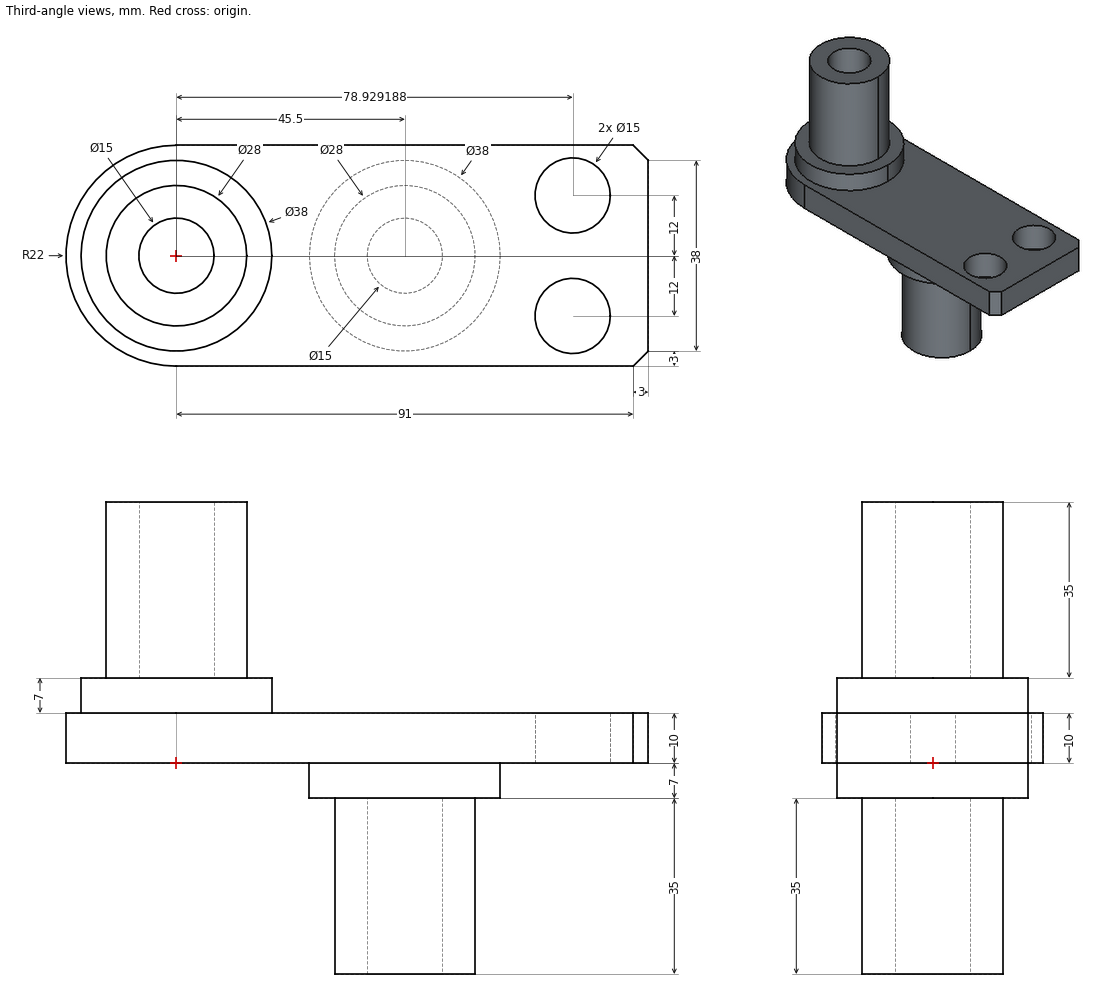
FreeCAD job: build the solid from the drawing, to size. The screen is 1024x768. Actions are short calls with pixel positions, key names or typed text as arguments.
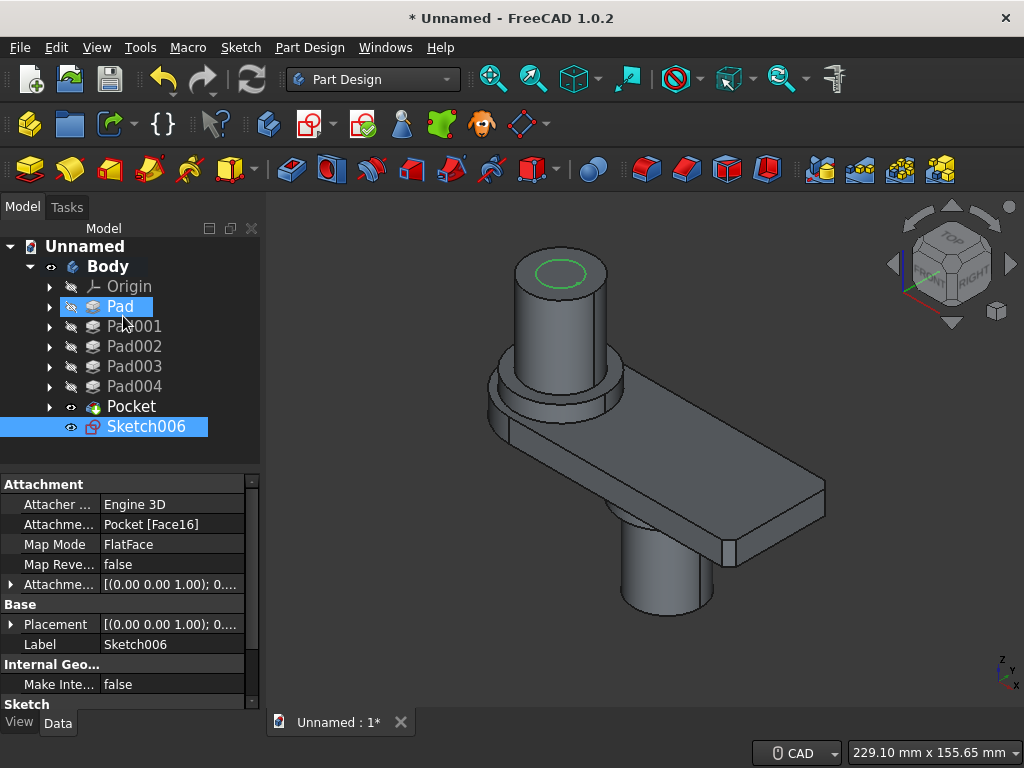
click(292, 170)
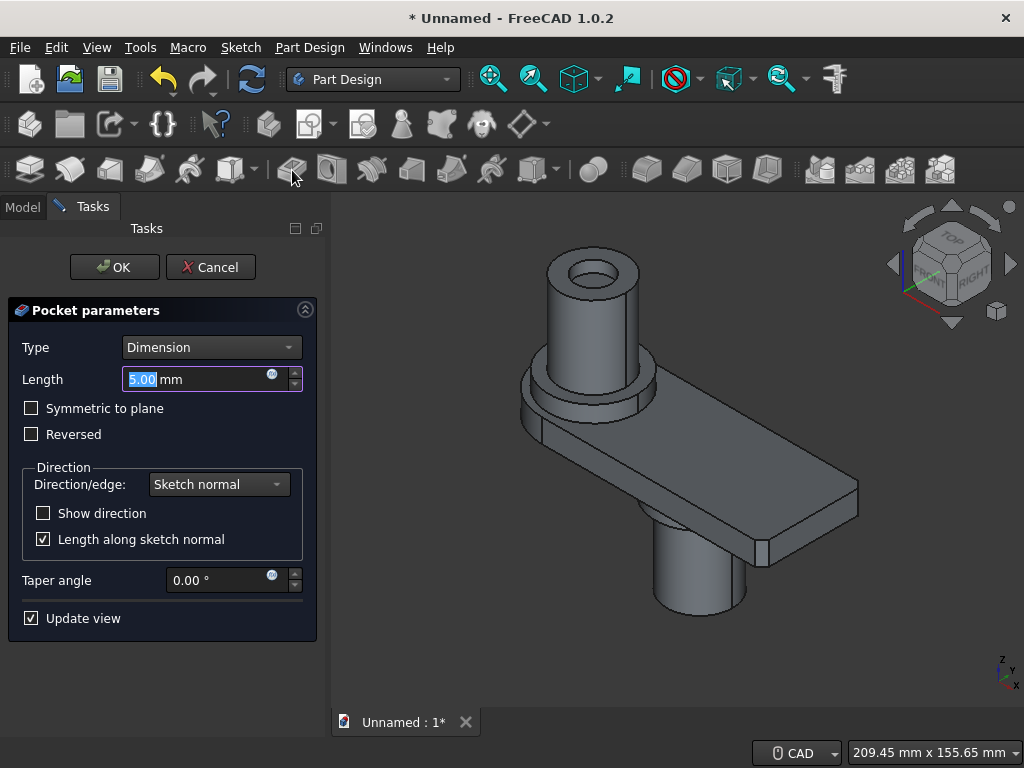
text(35)
key(Tab)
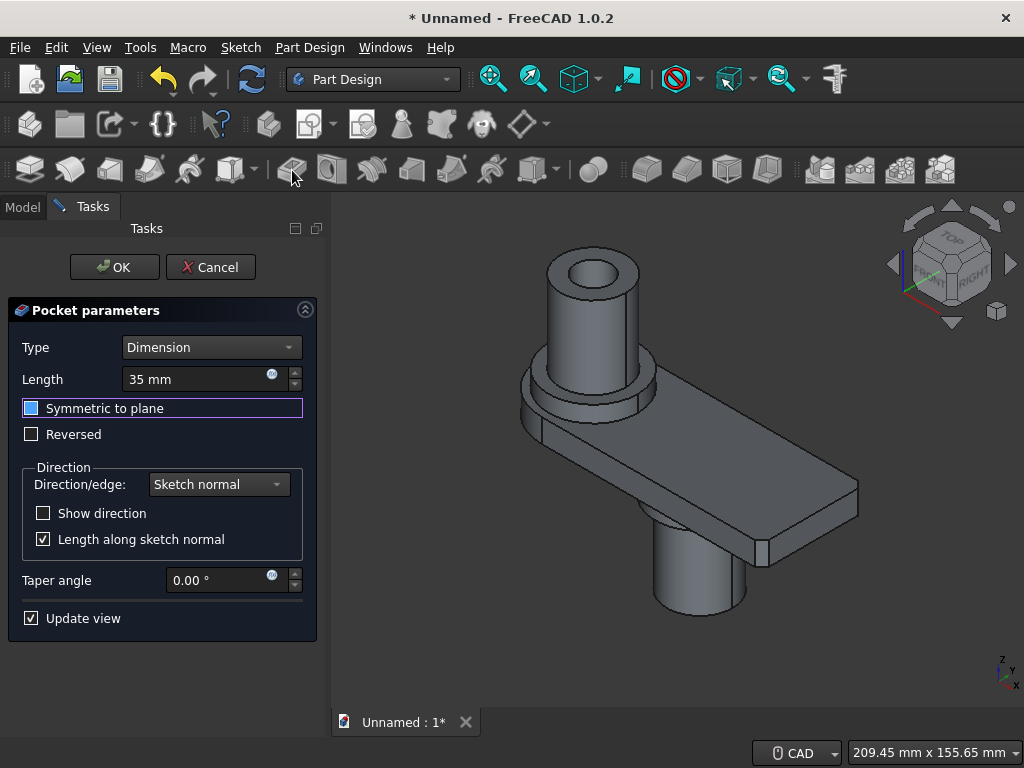
click(115, 267)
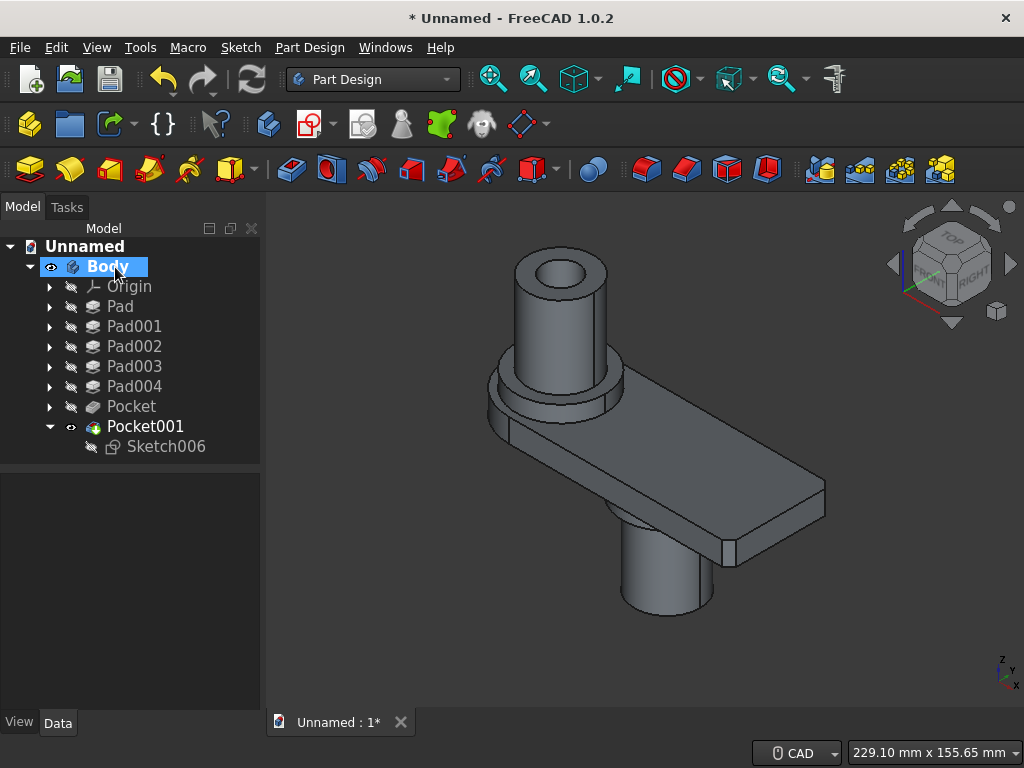
click(723, 480)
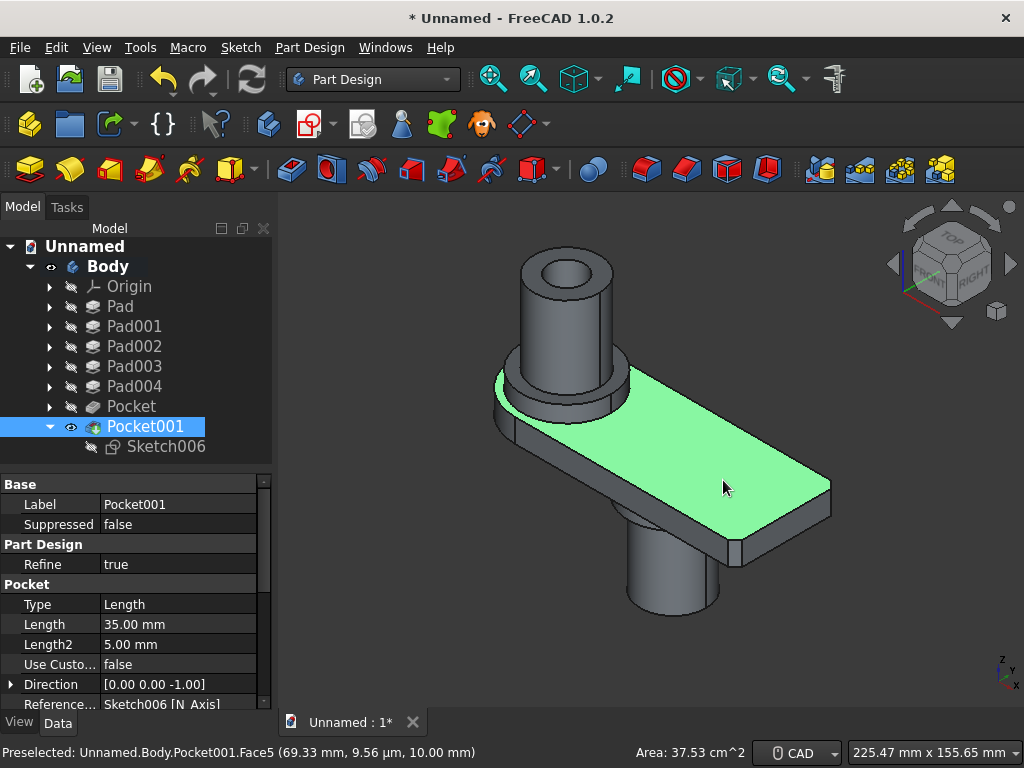
click(310, 124)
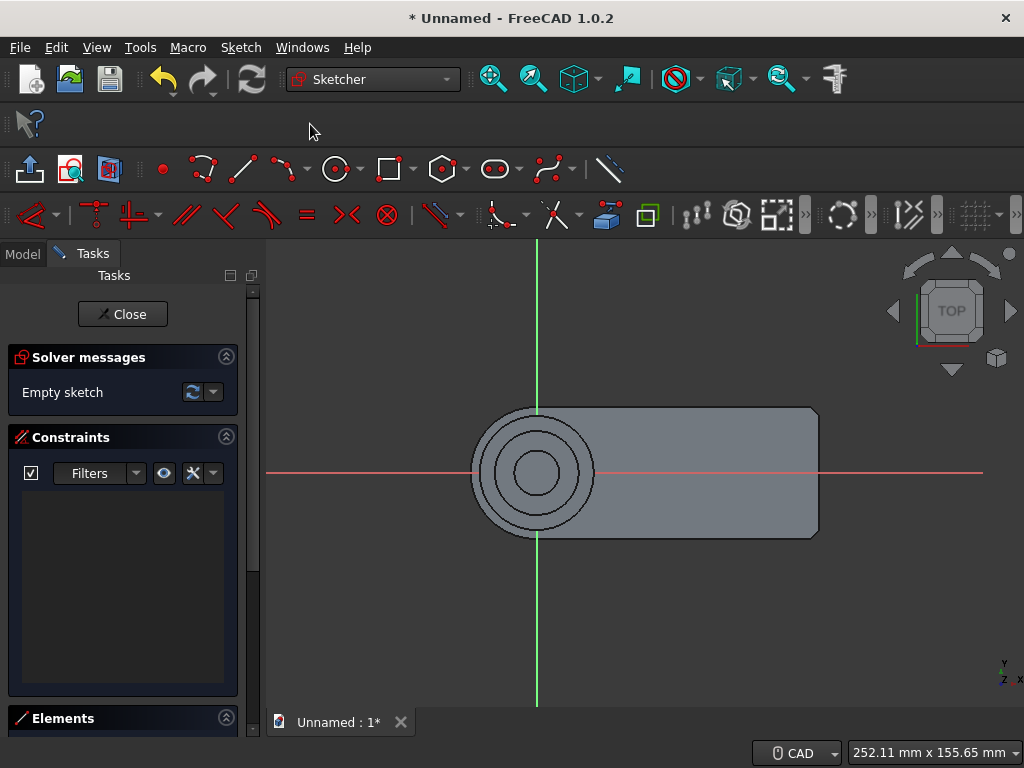
scroll(850, 473, up, 2)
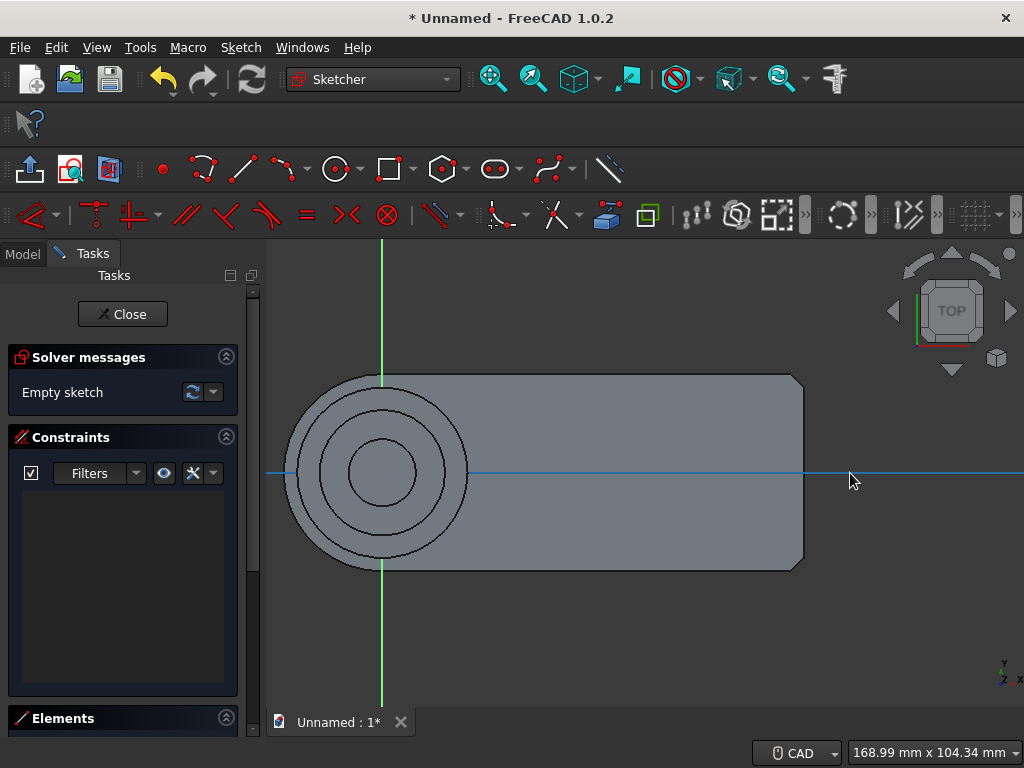
click(336, 170)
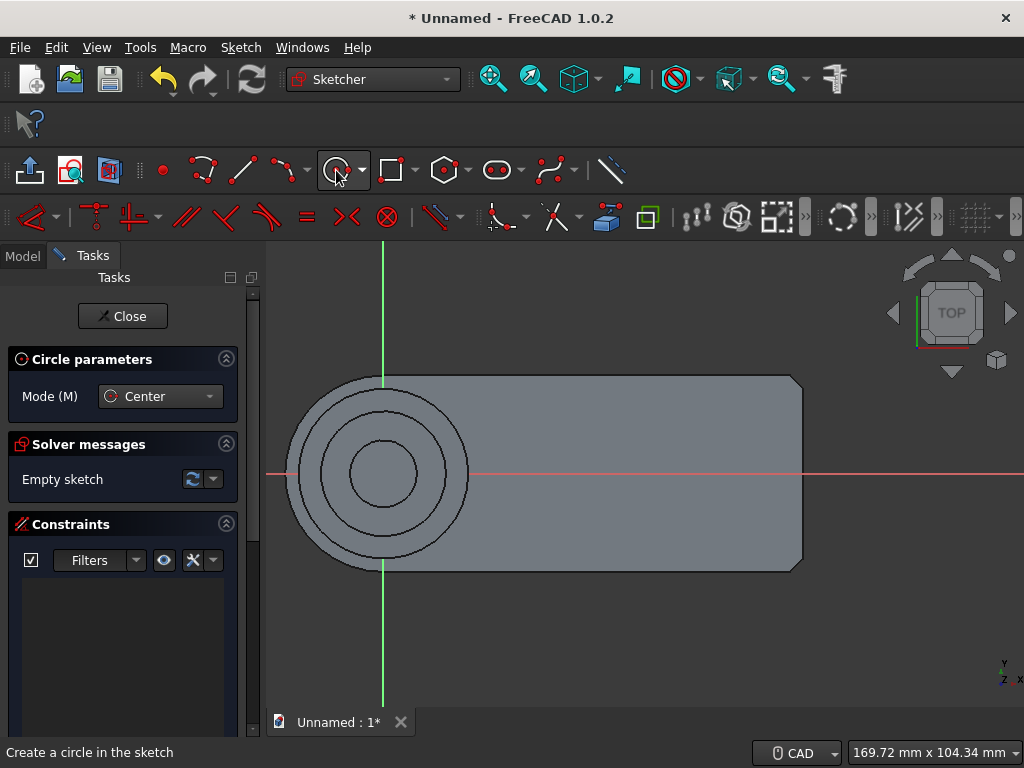
click(736, 420)
move(760, 396)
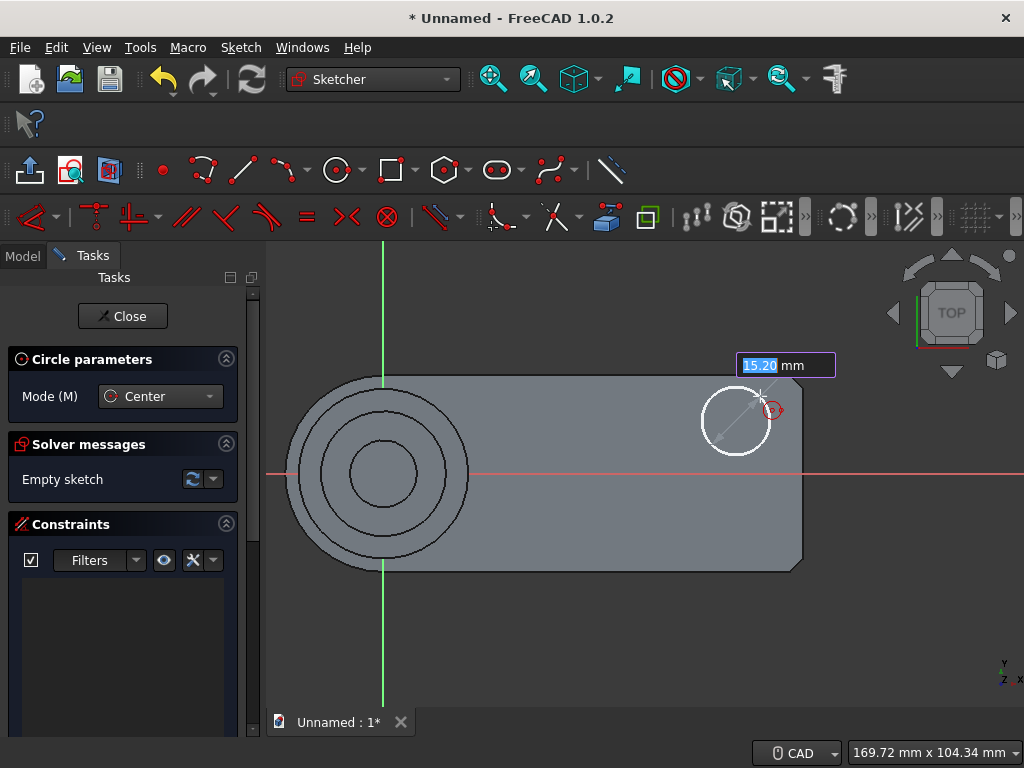
text(15)
key(Return)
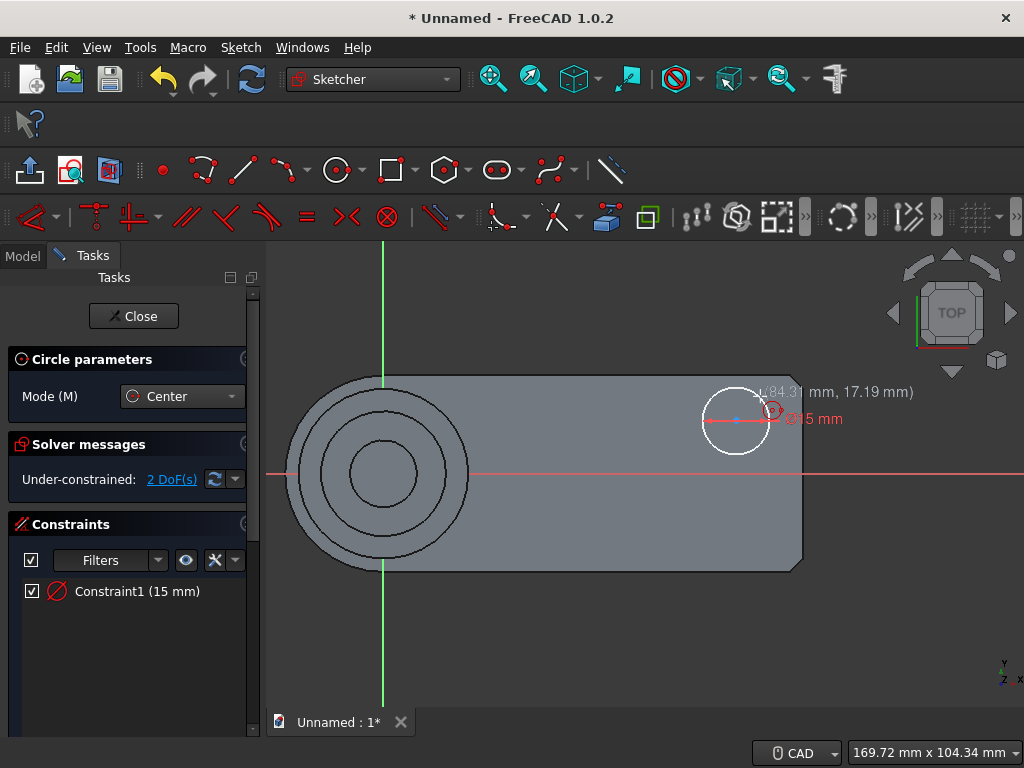
click(736, 527)
move(760, 504)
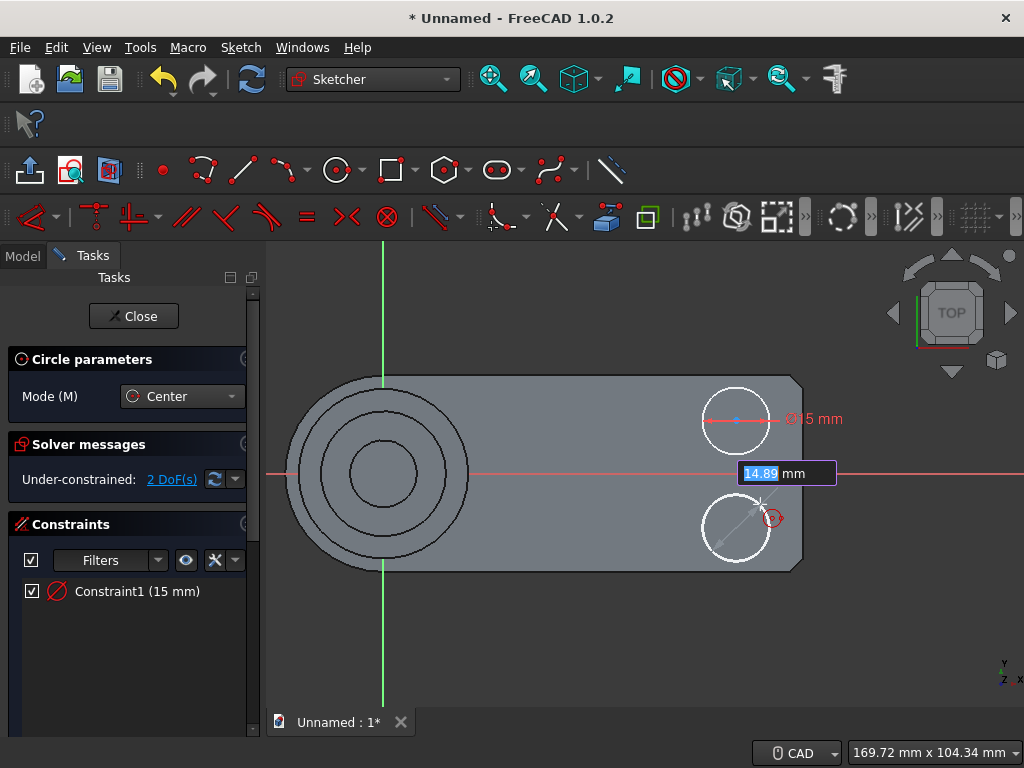
text(15)
key(Return)
key(Escape)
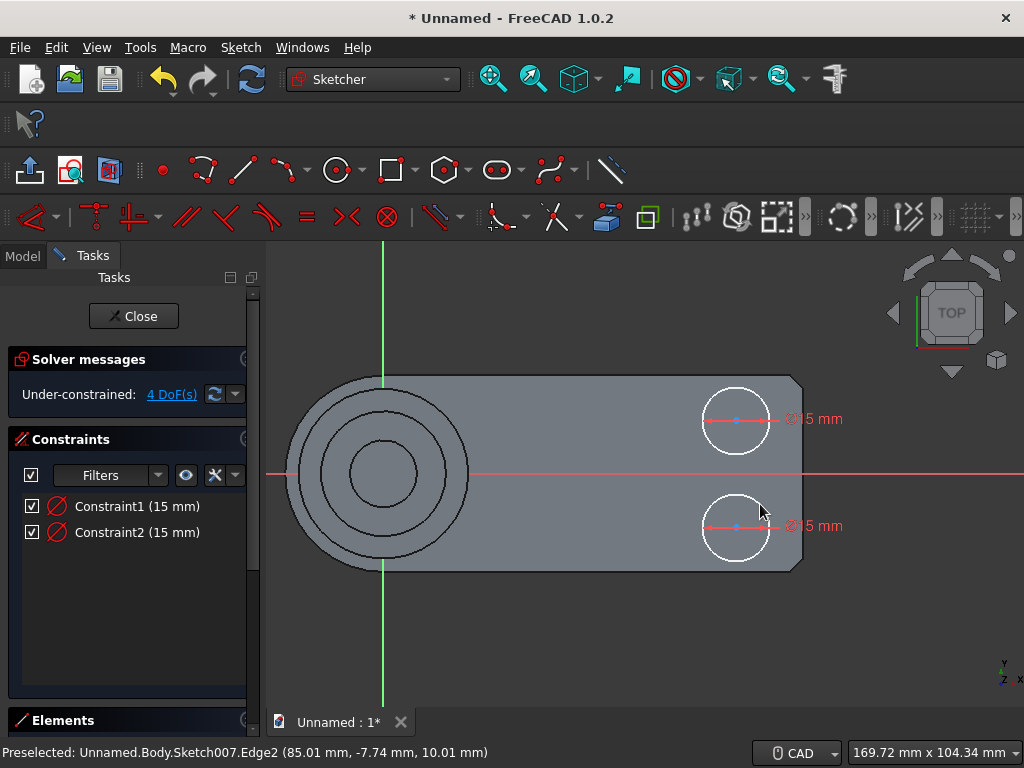
click(736, 421)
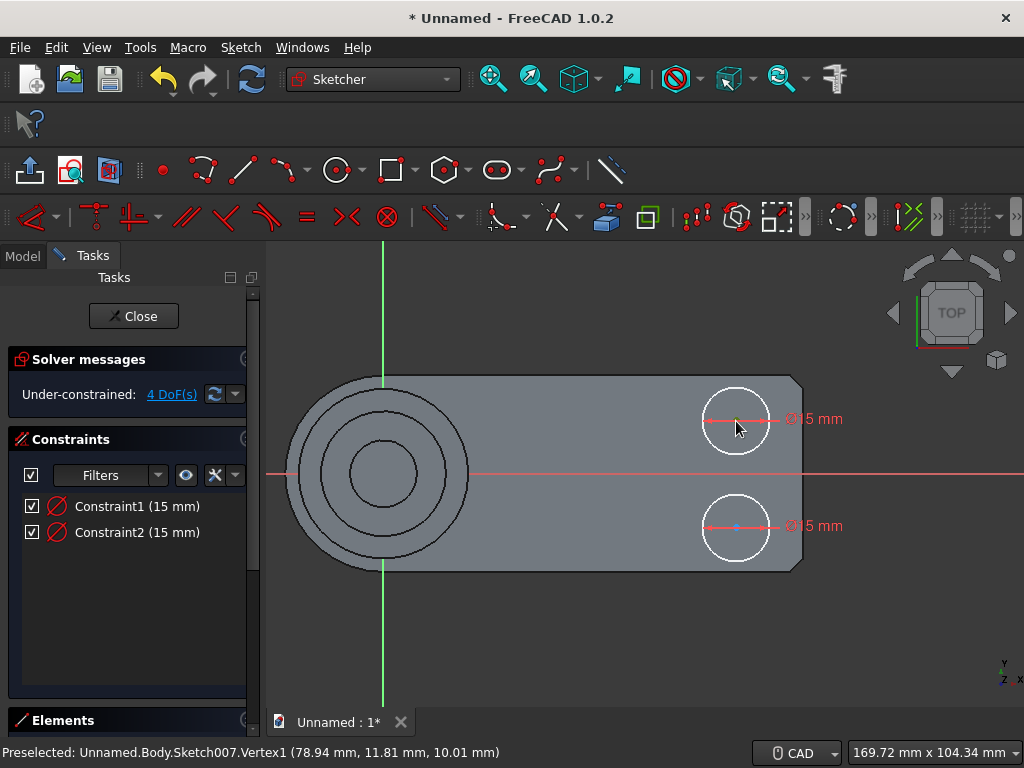
click(736, 528)